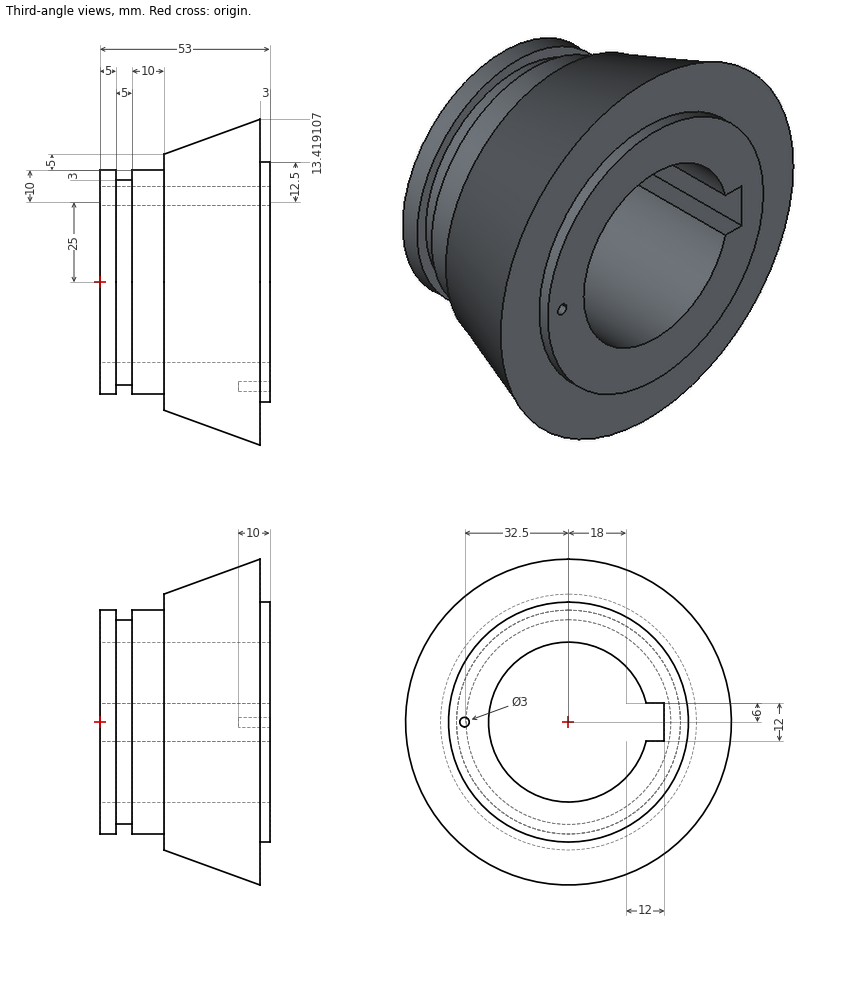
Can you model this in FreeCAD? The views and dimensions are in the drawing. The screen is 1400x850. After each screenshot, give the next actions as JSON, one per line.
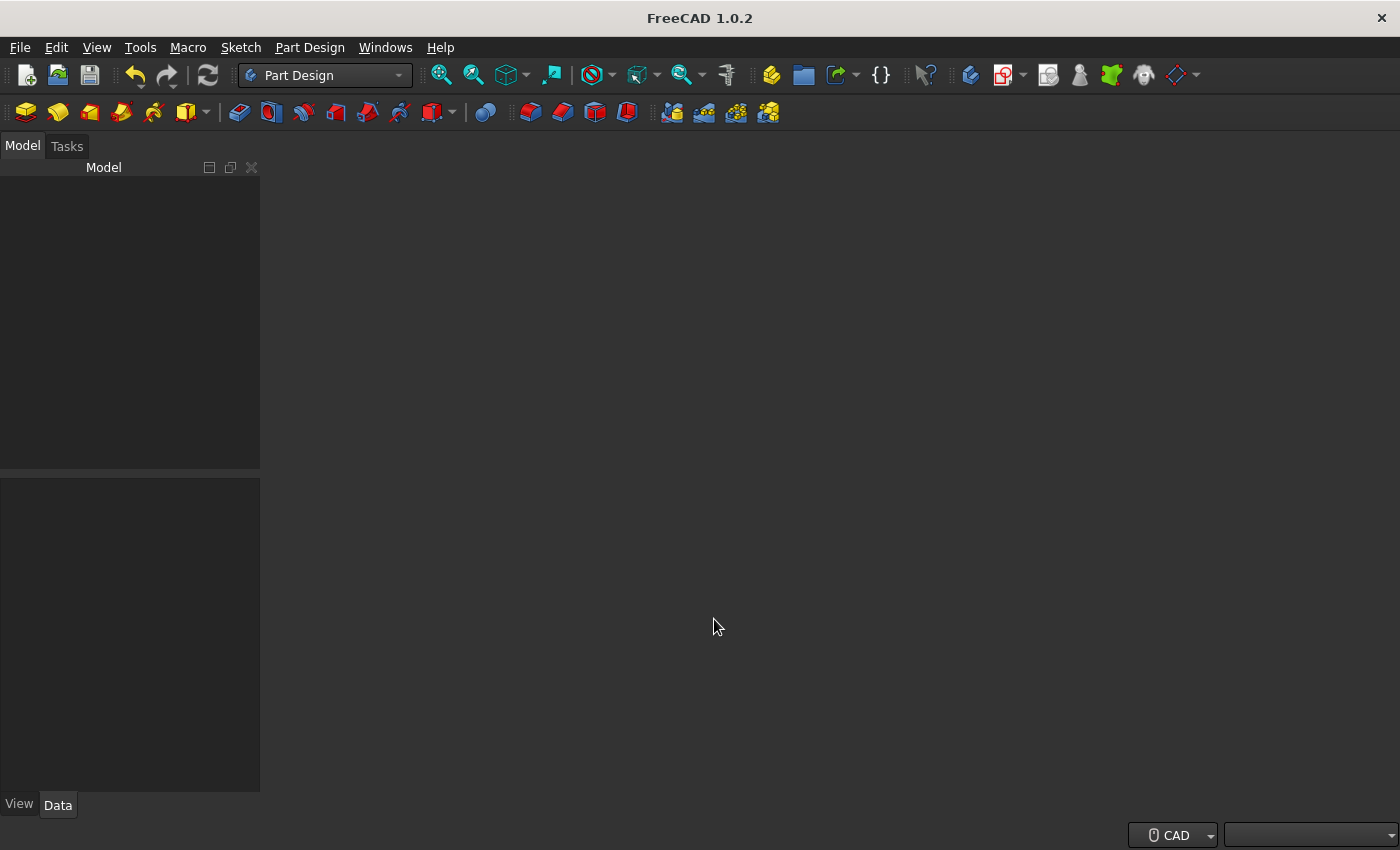
{"action": "left_click", "coordinate": [26, 76]}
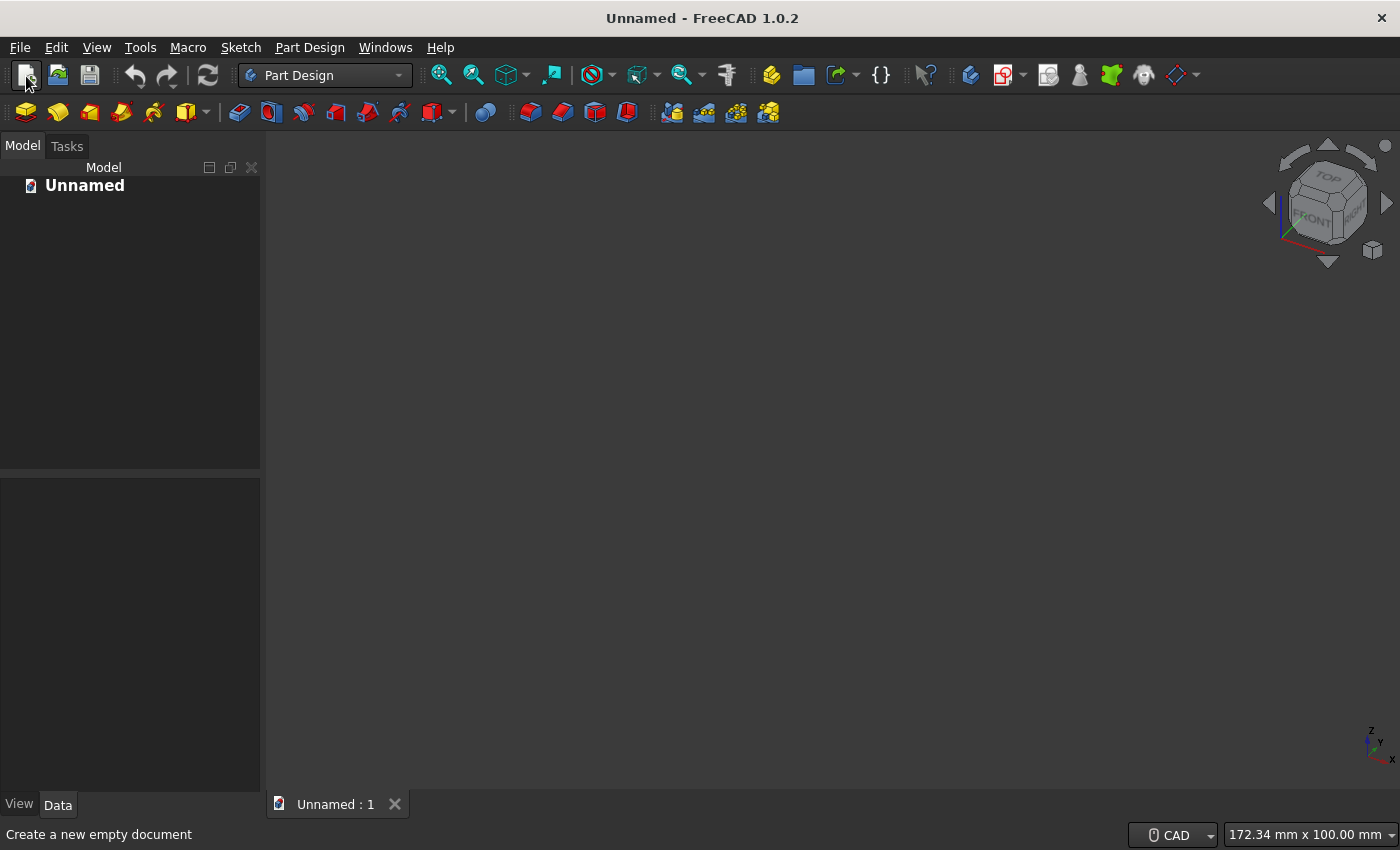
{"action": "left_click", "coordinate": [1004, 76]}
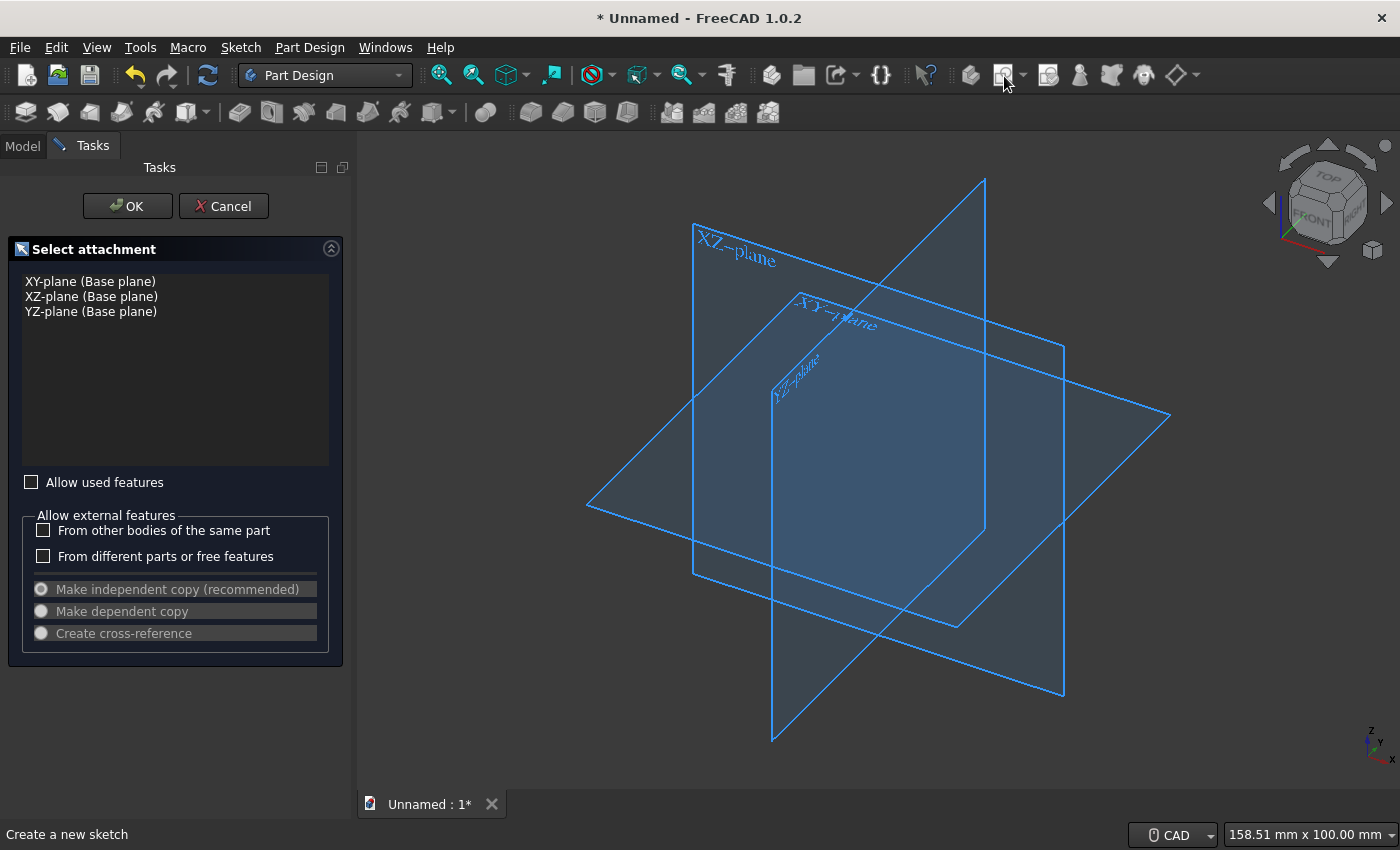
{"action": "left_click", "coordinate": [82, 282]}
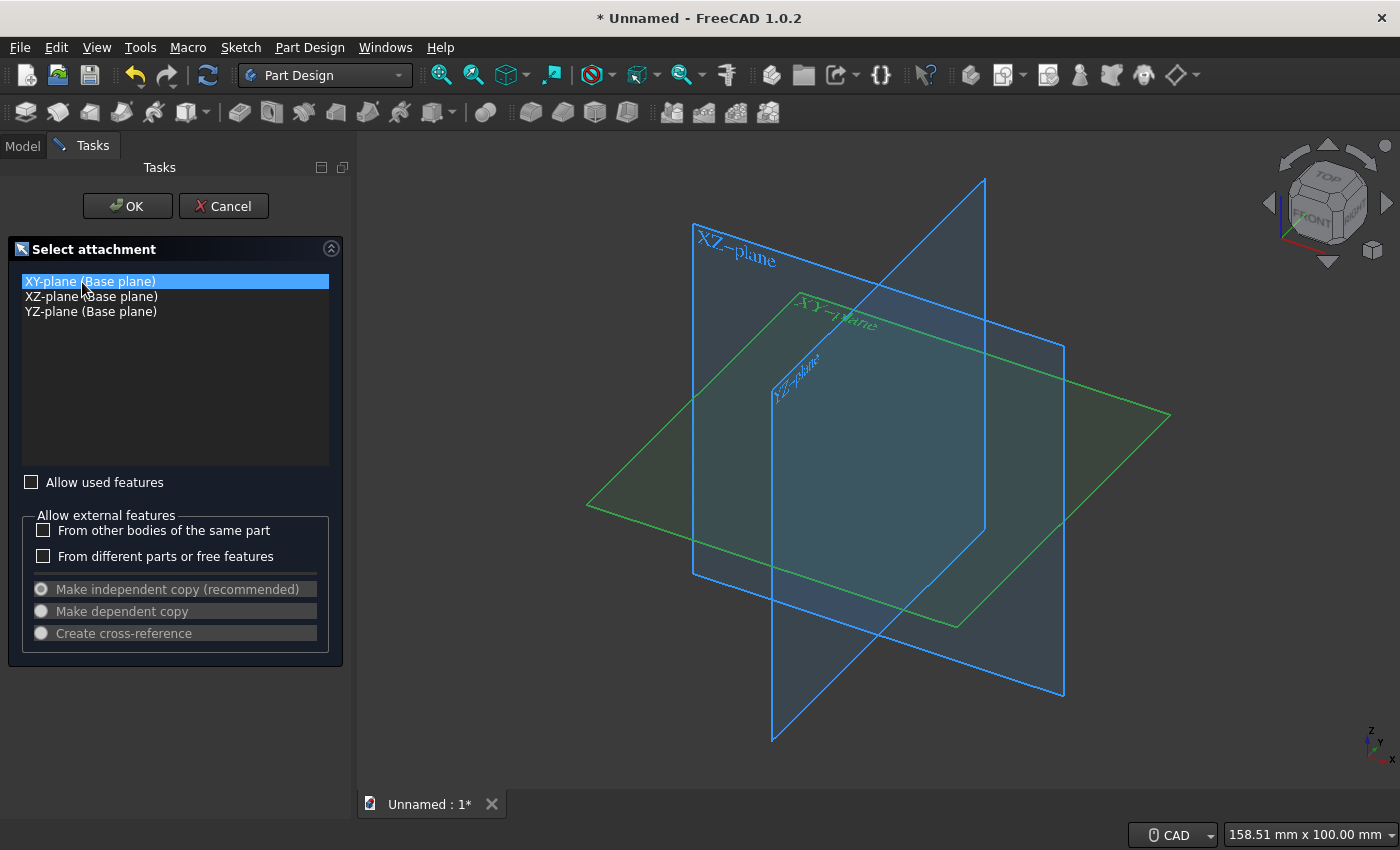
{"action": "left_click", "coordinate": [128, 206]}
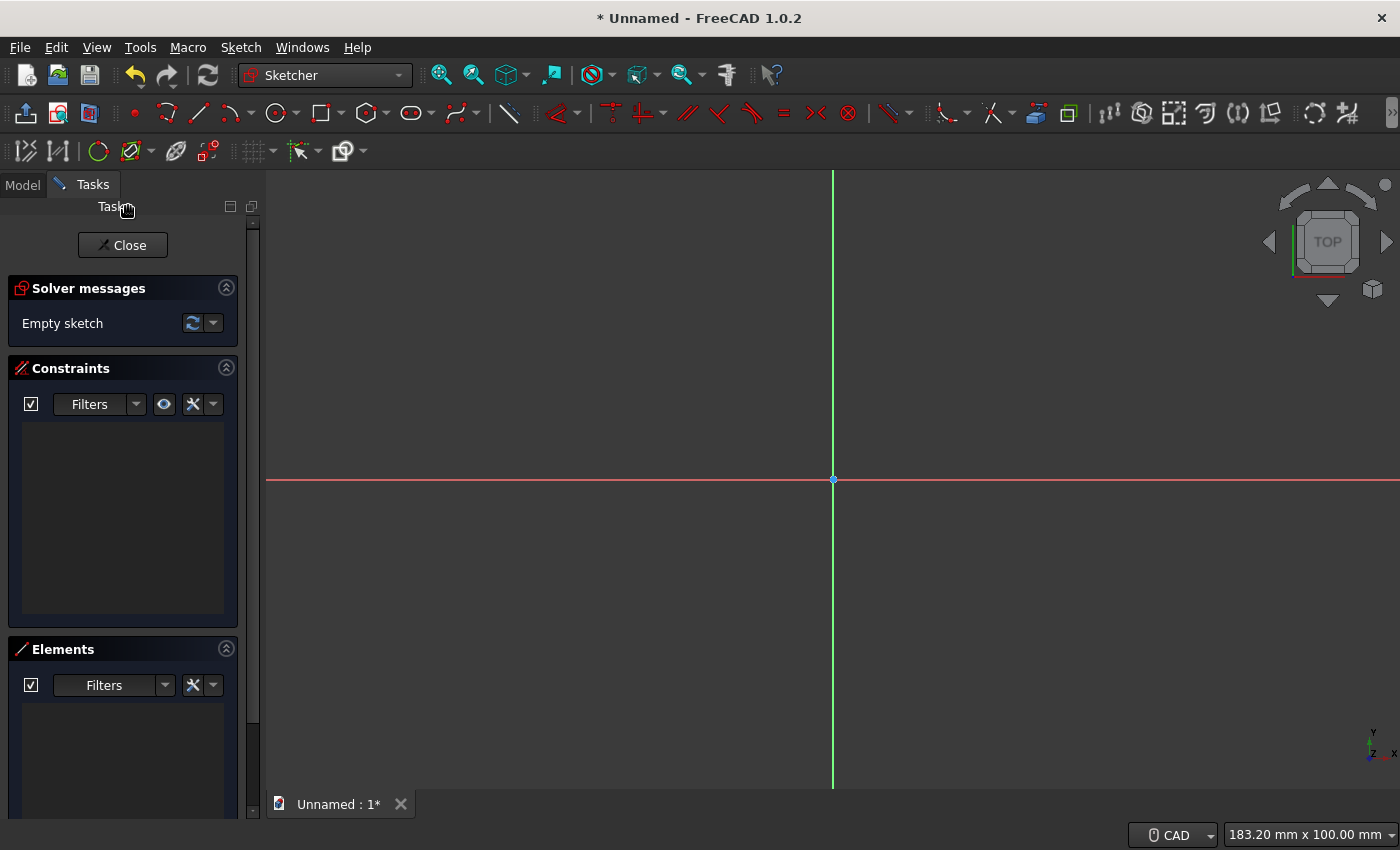
{"action": "scroll", "coordinate": [294, 761], "scroll_direction": "down", "scroll_amount": 1}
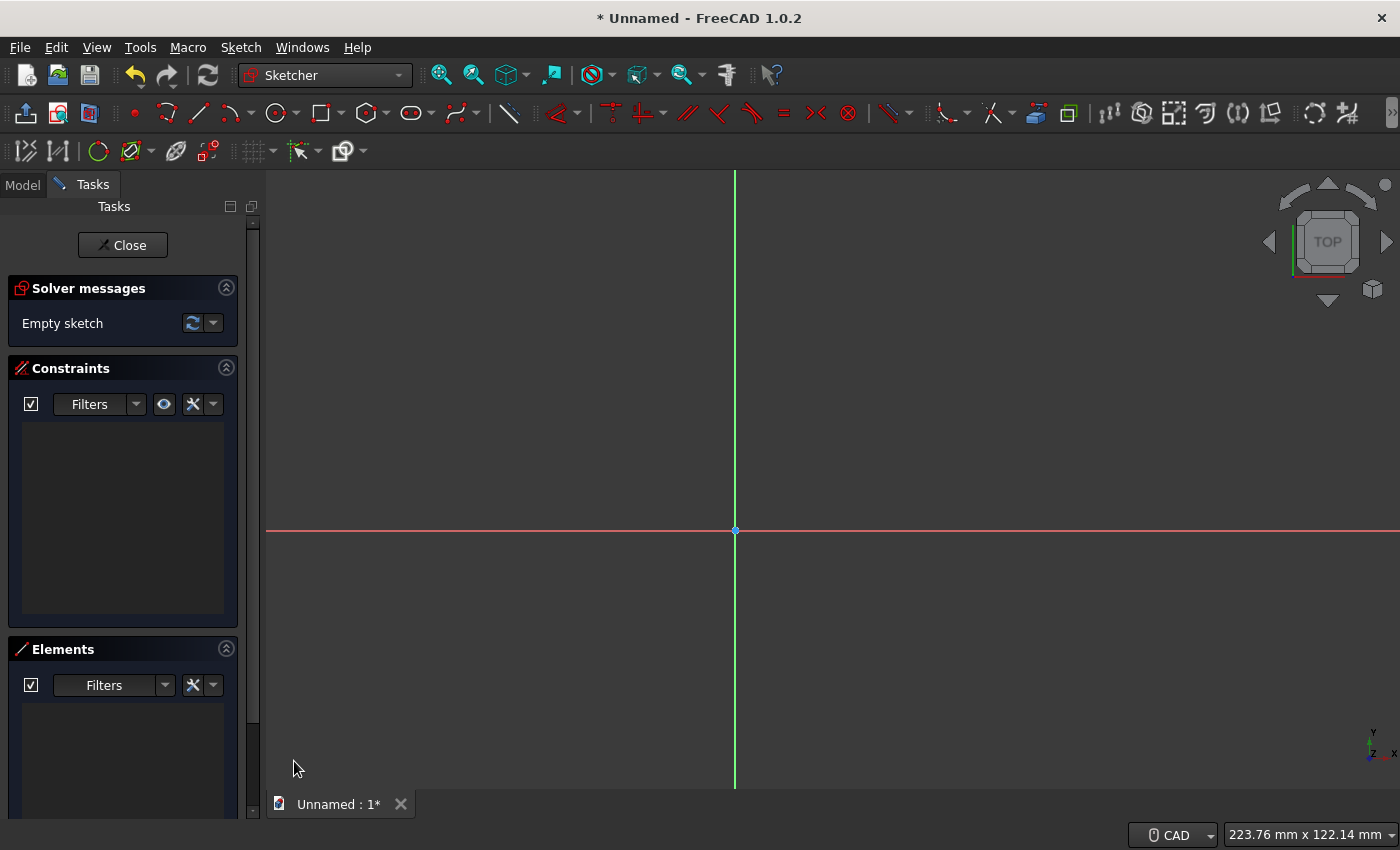
{"action": "scroll", "coordinate": [1083, 243], "scroll_direction": "up", "scroll_amount": 2}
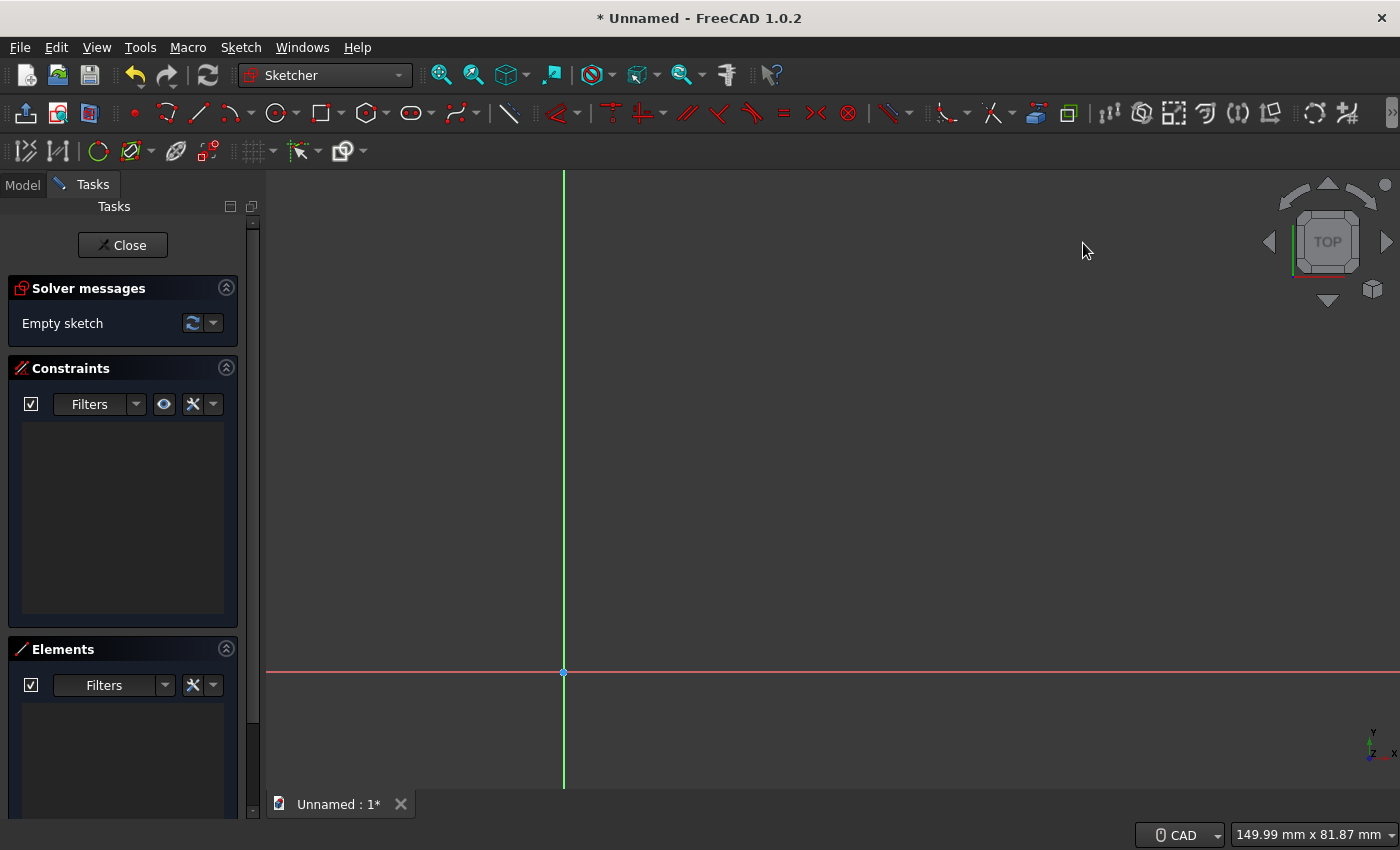
{"action": "left_click", "coordinate": [168, 114]}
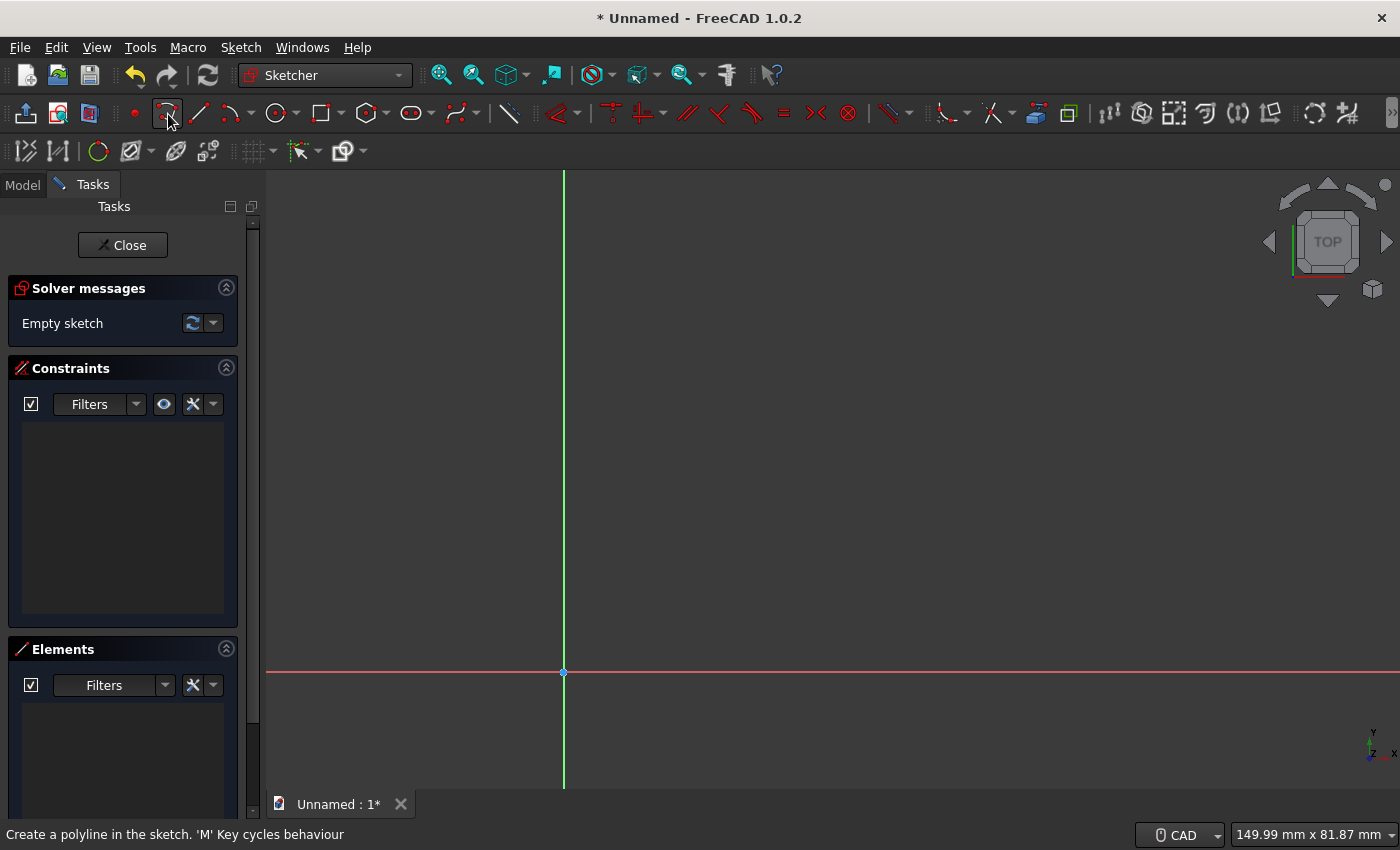
{"action": "left_click", "coordinate": [564, 483]}
{"action": "left_click", "coordinate": [965, 483]}
{"action": "left_click", "coordinate": [965, 389]}
{"action": "left_click", "coordinate": [942, 389]}
{"action": "left_click", "coordinate": [942, 287]}
{"action": "left_click", "coordinate": [715, 370]}
{"action": "left_click", "coordinate": [715, 408]}
{"action": "left_click", "coordinate": [640, 408]}
{"action": "left_click", "coordinate": [640, 430]}
{"action": "left_click", "coordinate": [602, 430]}
{"action": "left_click", "coordinate": [602, 408]}
{"action": "left_click", "coordinate": [573, 408]}
{"action": "left_click", "coordinate": [564, 484]}
{"action": "key", "text": "Escape"}
{"action": "key", "text": "Escape"}